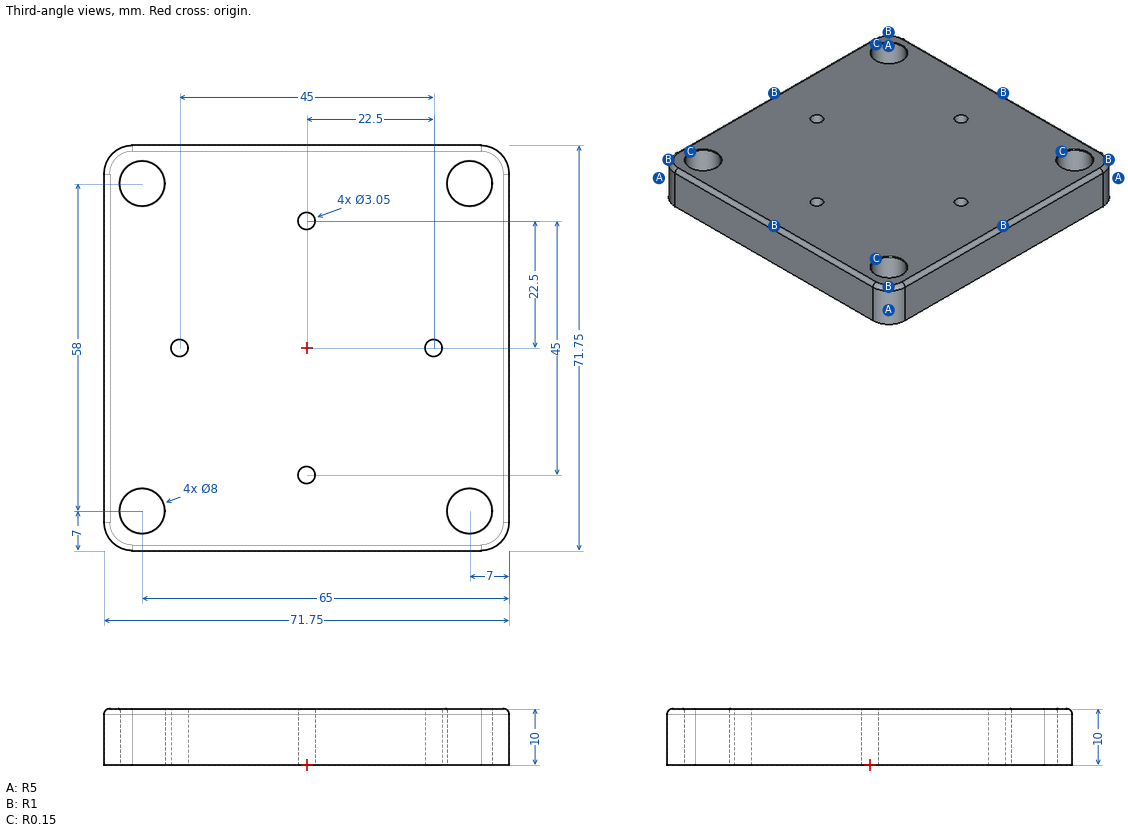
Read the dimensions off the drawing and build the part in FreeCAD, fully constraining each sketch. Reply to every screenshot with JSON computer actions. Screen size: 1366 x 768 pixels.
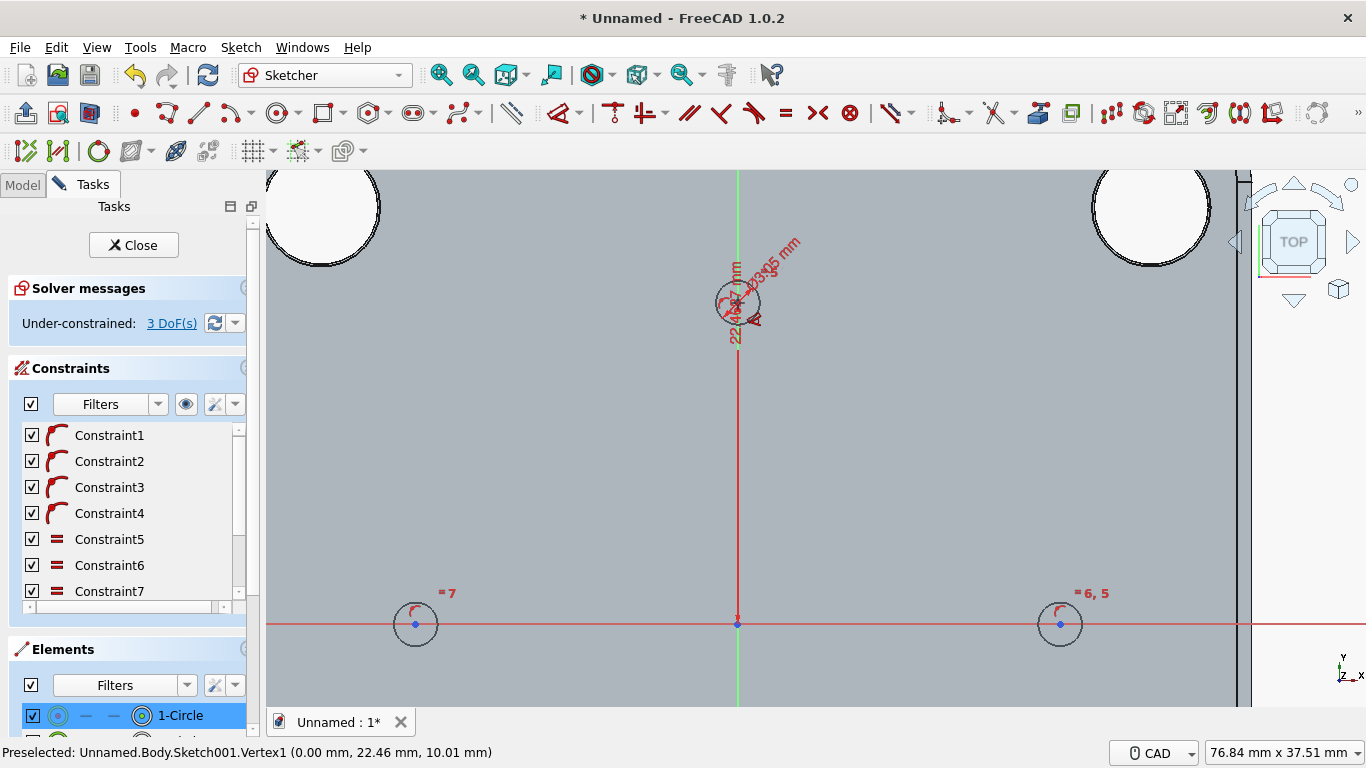
{"action": "scroll", "coordinate": [755, 287], "scroll_direction": "down", "scroll_amount": 4}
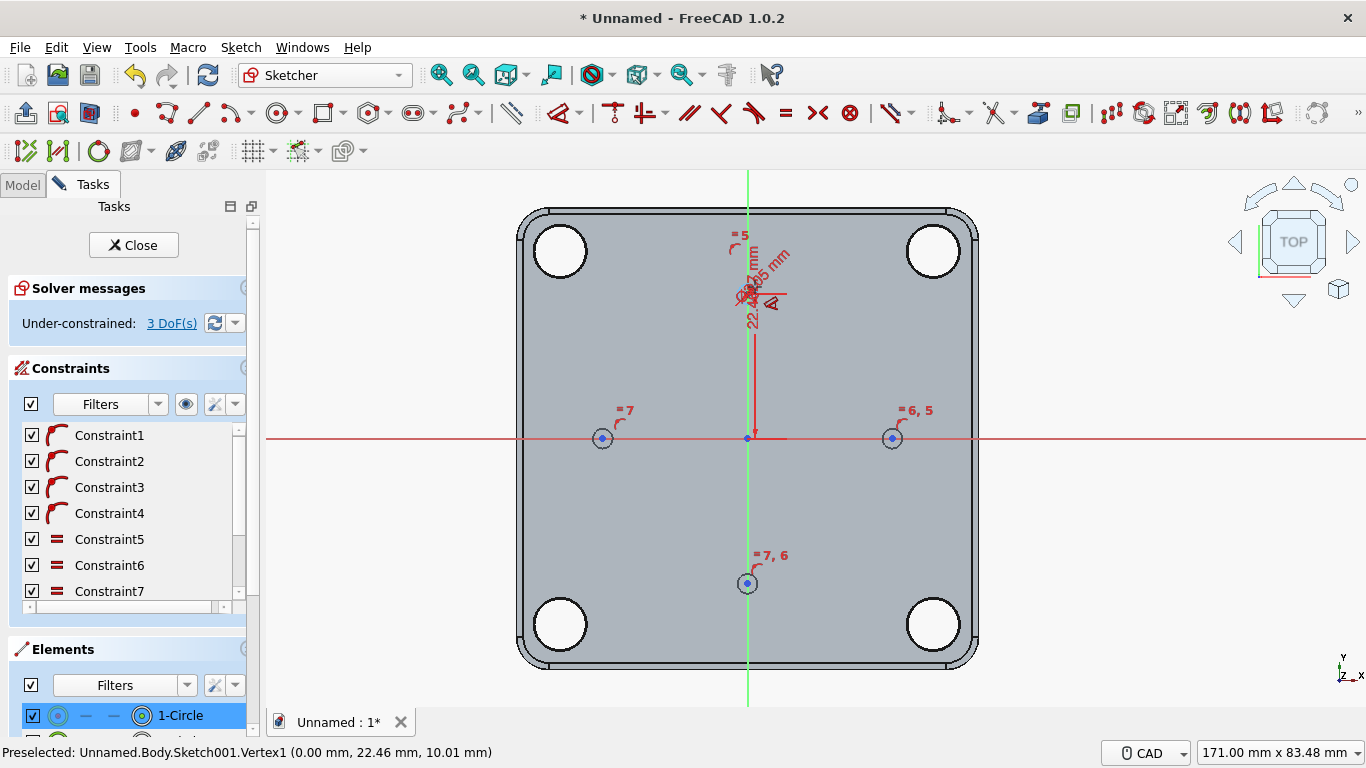
{"action": "left_click", "coordinate": [748, 584]}
{"action": "left_click", "coordinate": [782, 372]}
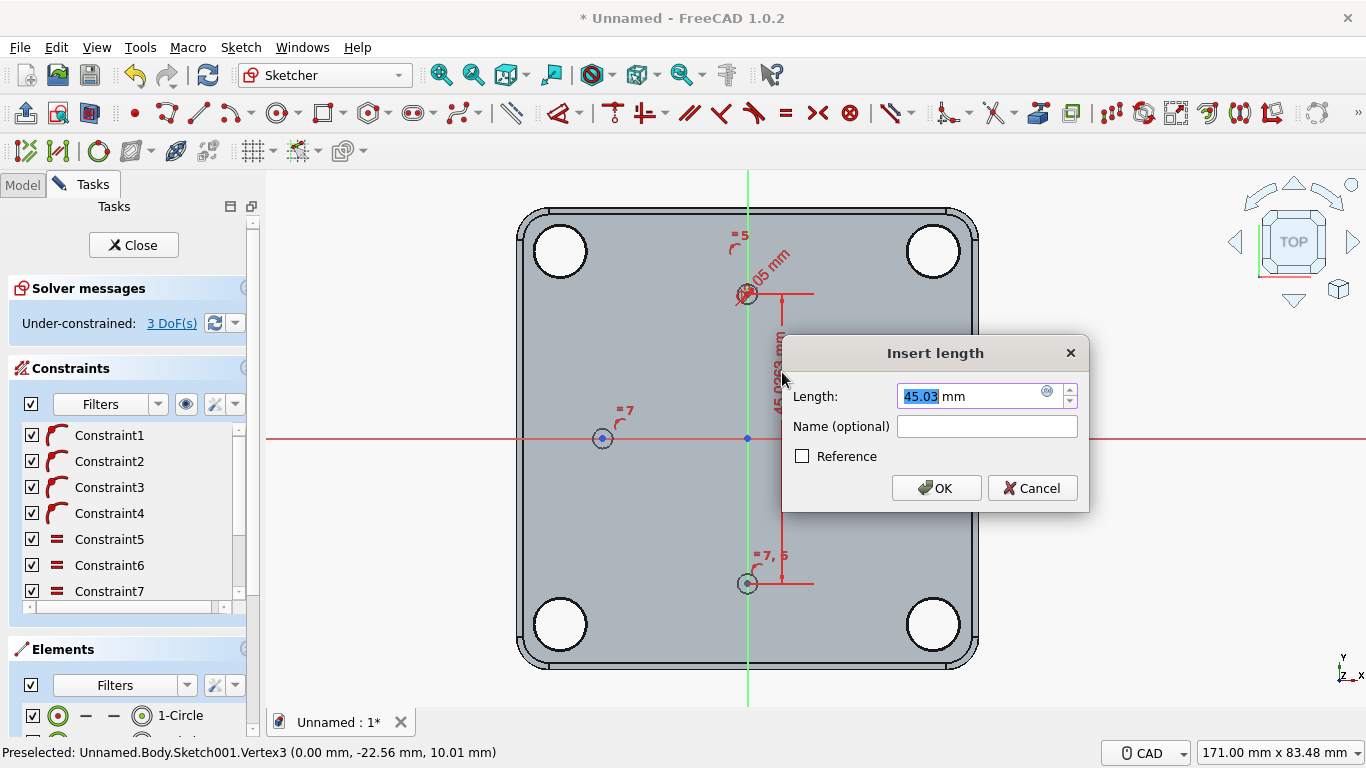
{"action": "type", "text": "45"}
{"action": "key", "text": "Return"}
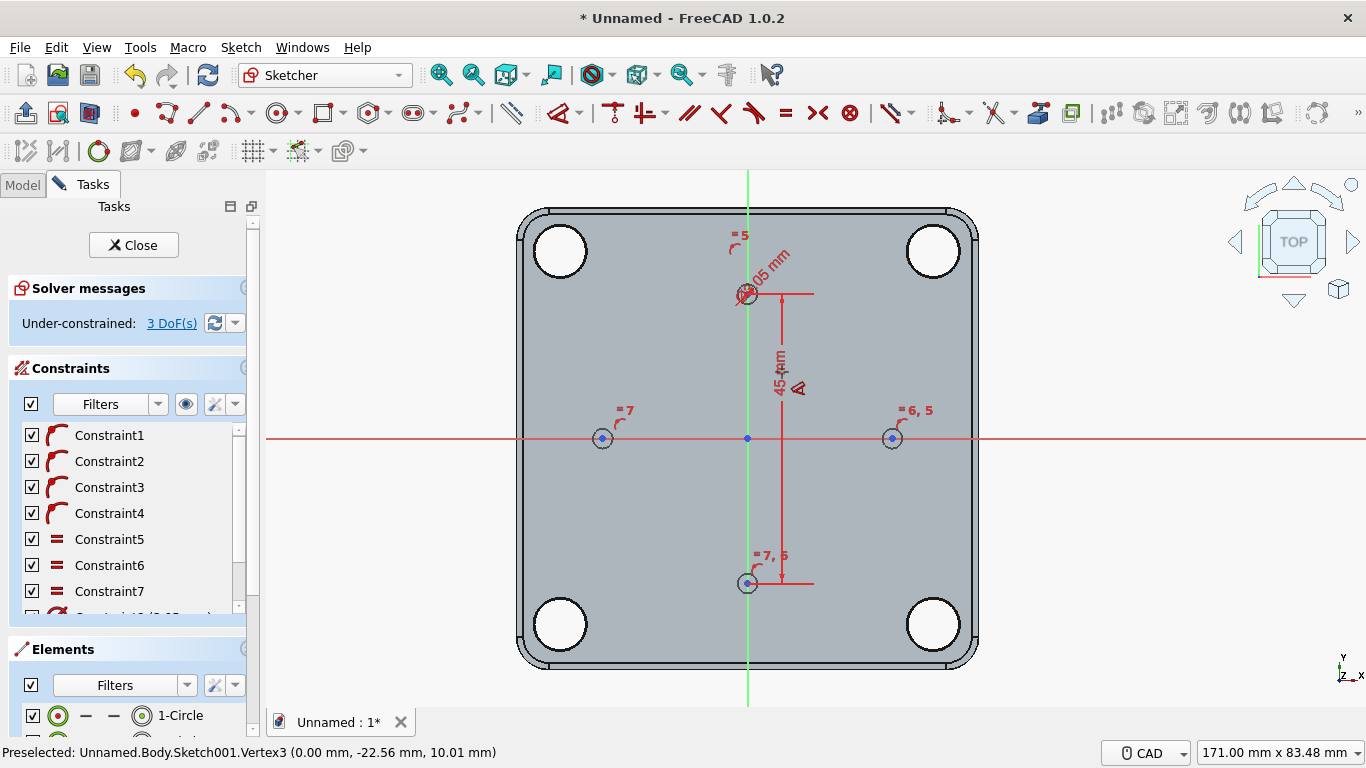
{"action": "left_click", "coordinate": [892, 439]}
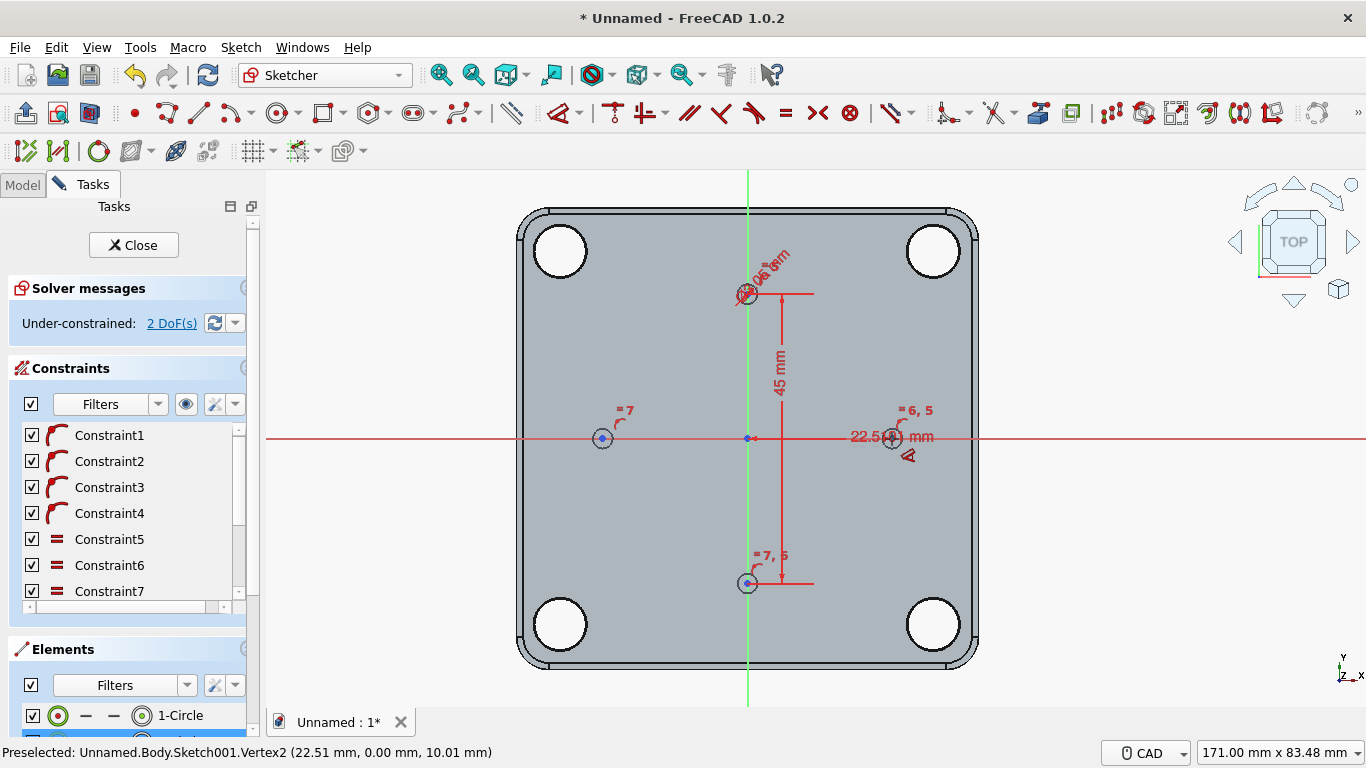
{"action": "left_click", "coordinate": [603, 439]}
{"action": "left_click", "coordinate": [681, 473]}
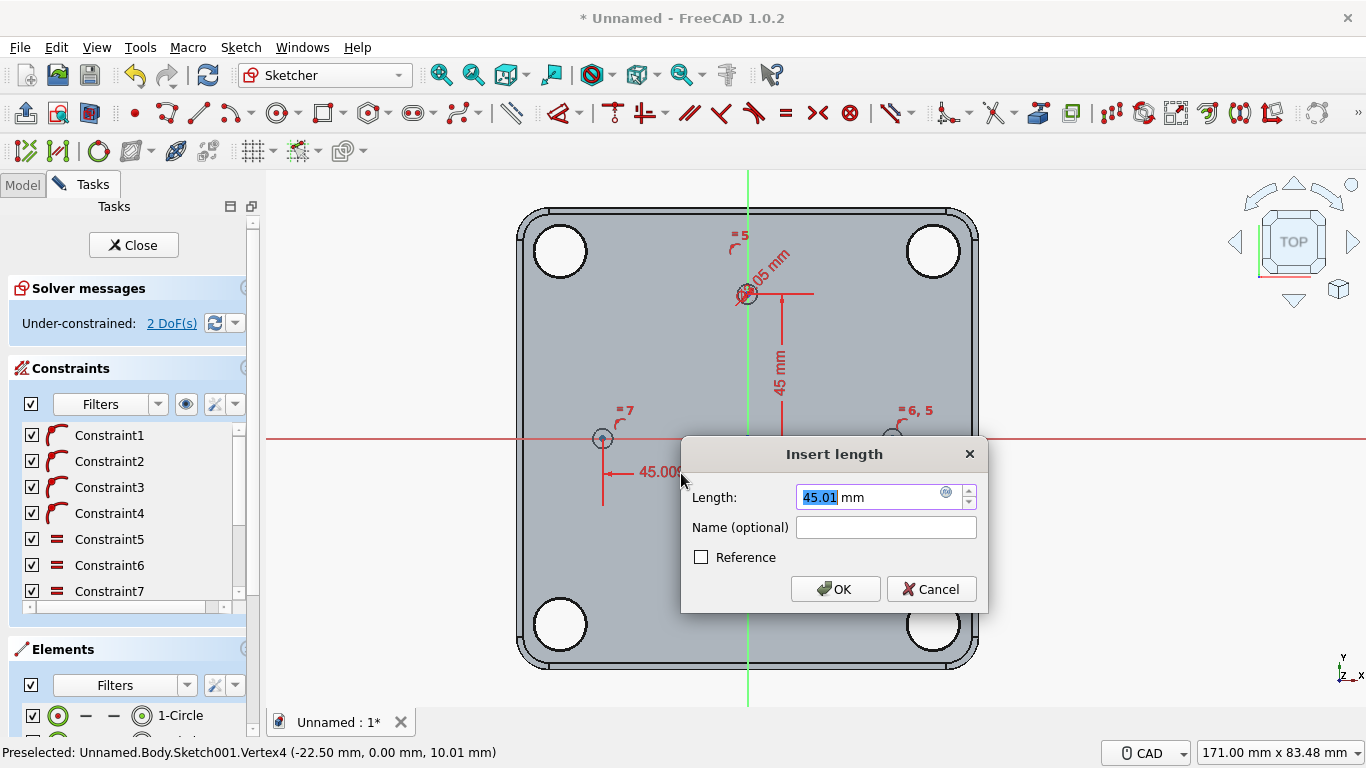
{"action": "type", "text": "45"}
{"action": "key", "text": "Return"}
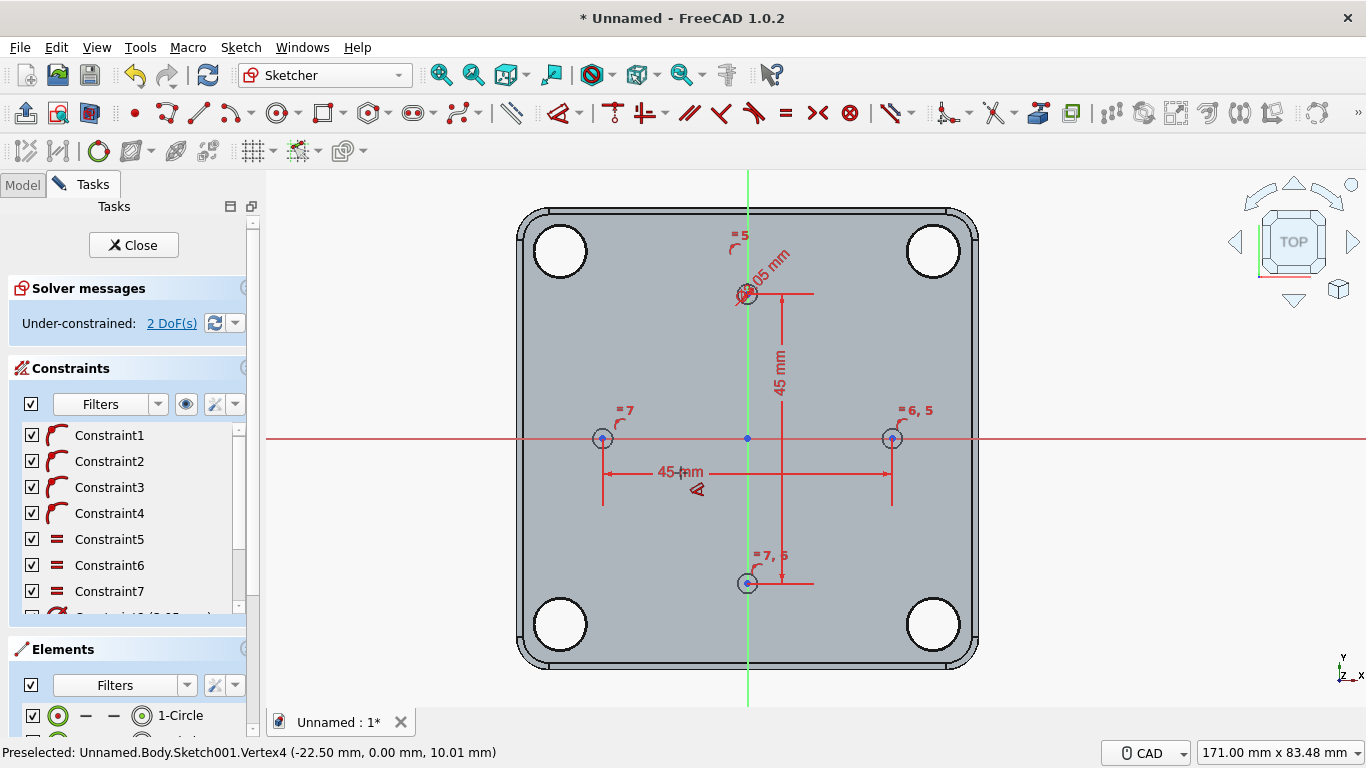
{"action": "left_click", "coordinate": [748, 294]}
{"action": "left_click", "coordinate": [782, 333]}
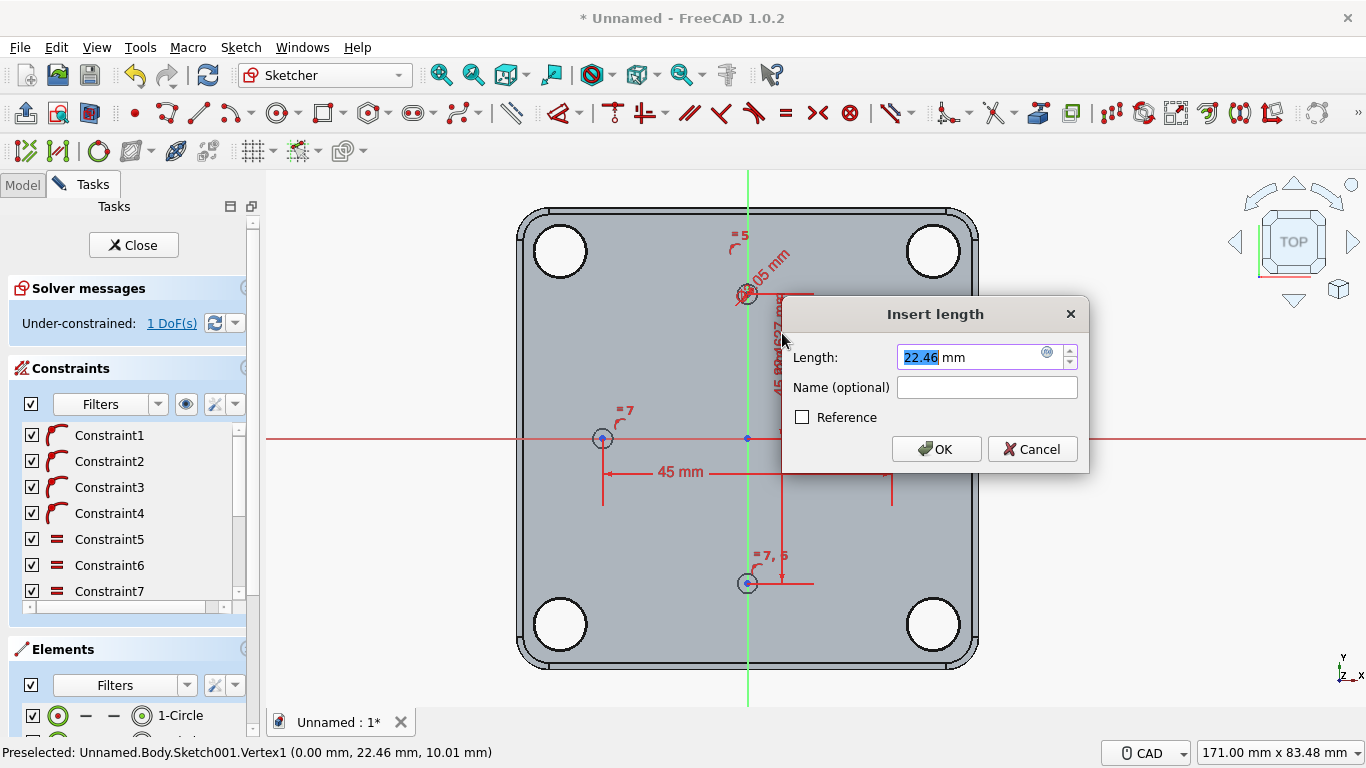
{"action": "type", "text": "22.5"}
{"action": "key", "text": "Return"}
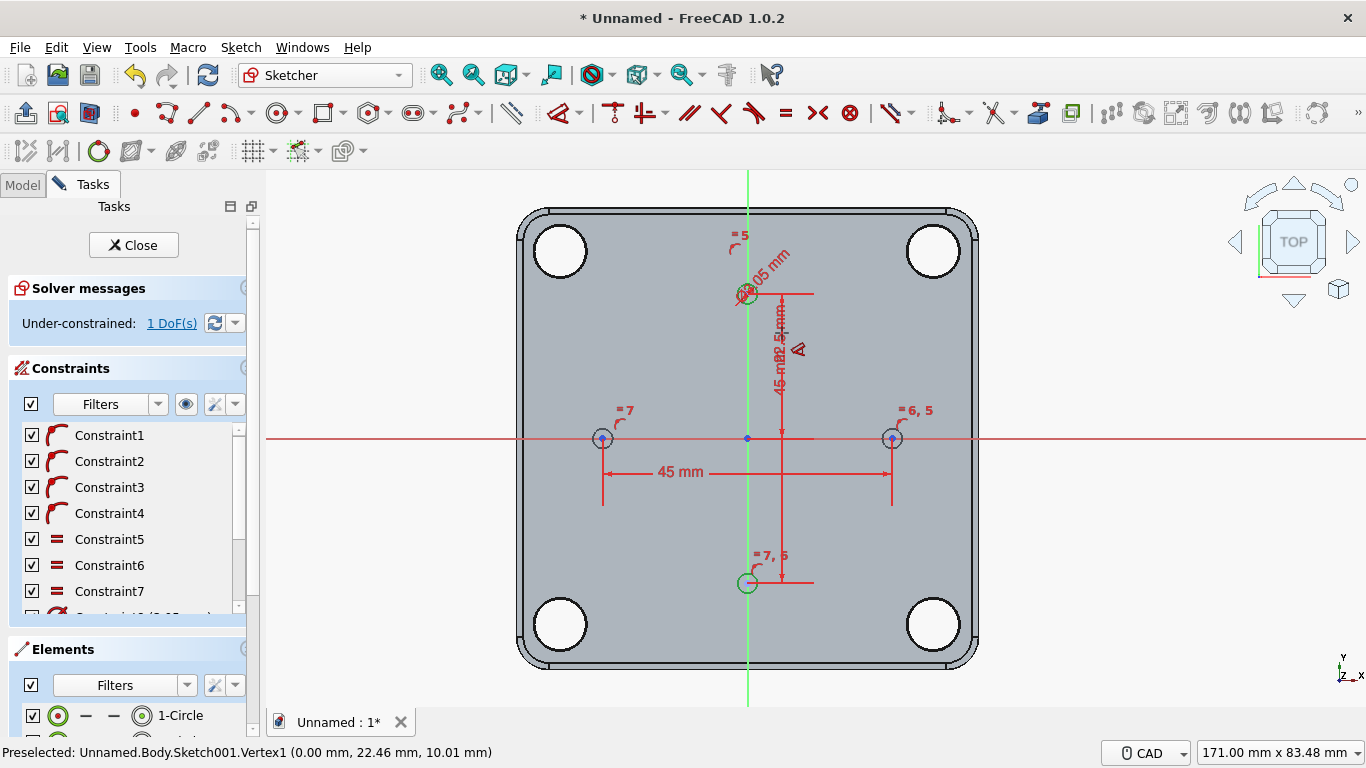
{"action": "left_click", "coordinate": [892, 439]}
{"action": "left_click", "coordinate": [820, 473]}